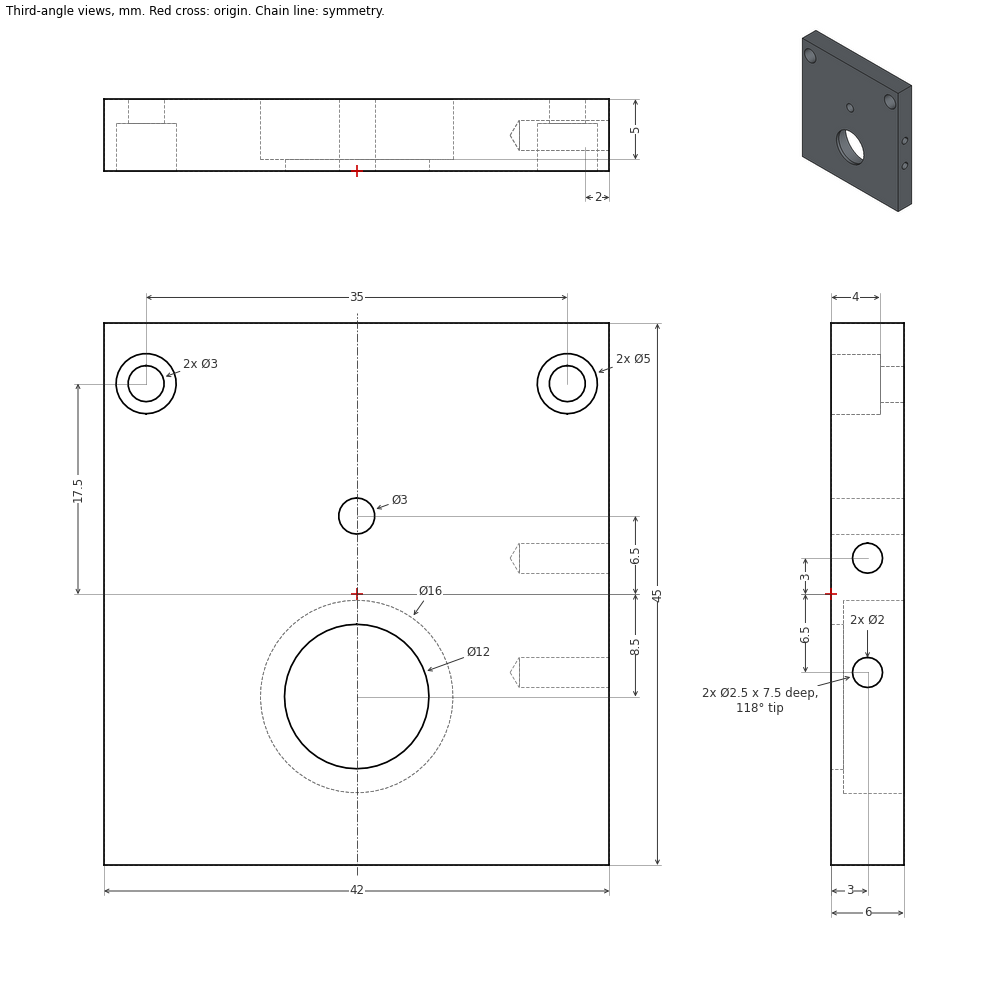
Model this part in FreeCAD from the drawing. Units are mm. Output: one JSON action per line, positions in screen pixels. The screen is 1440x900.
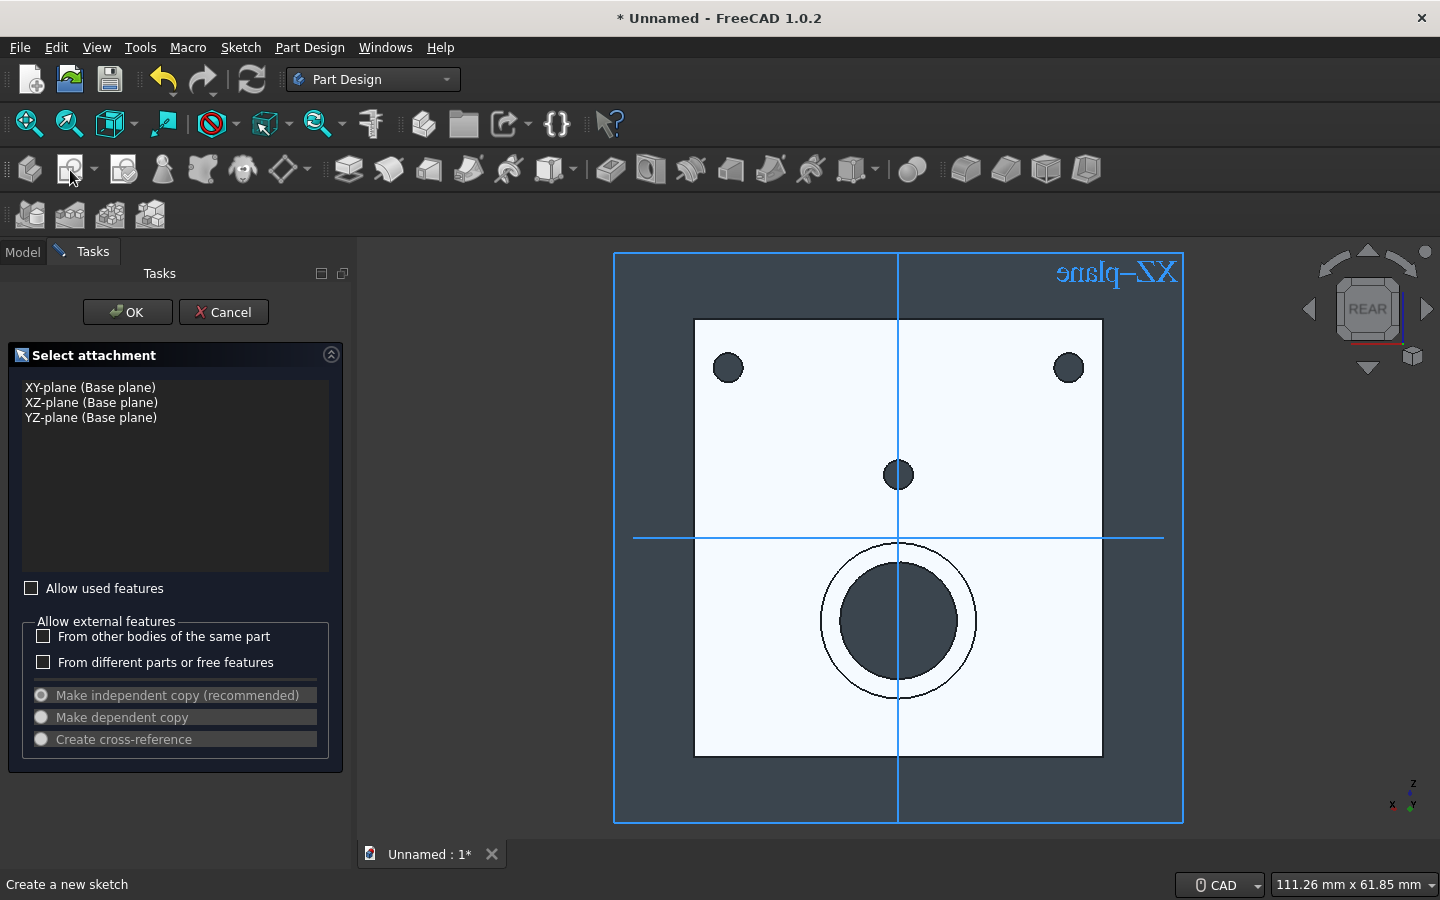
{"action": "left_click", "coordinate": [82, 402]}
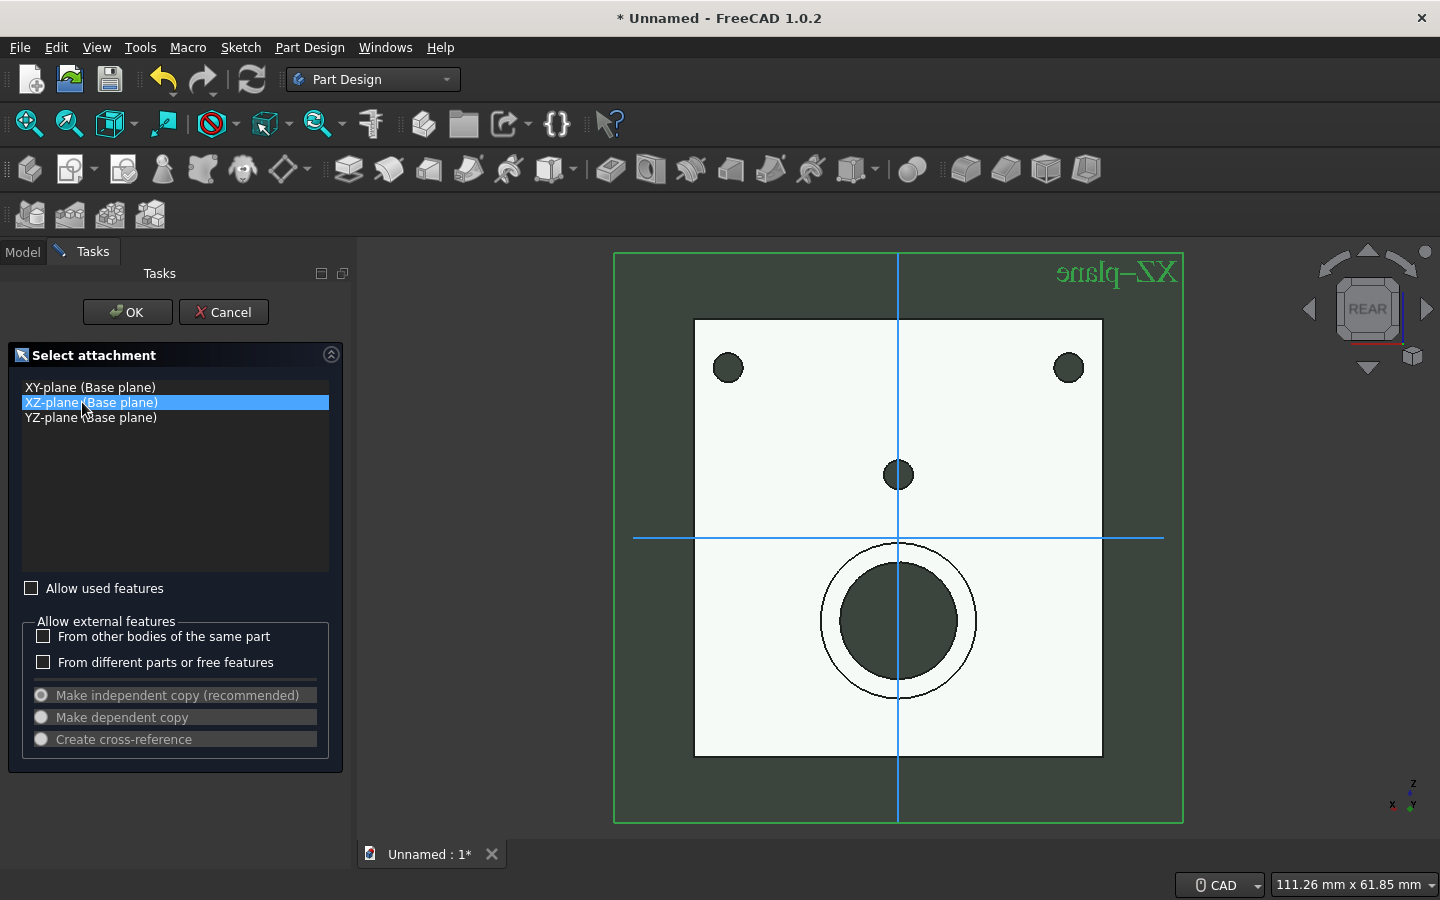
{"action": "left_click", "coordinate": [128, 312]}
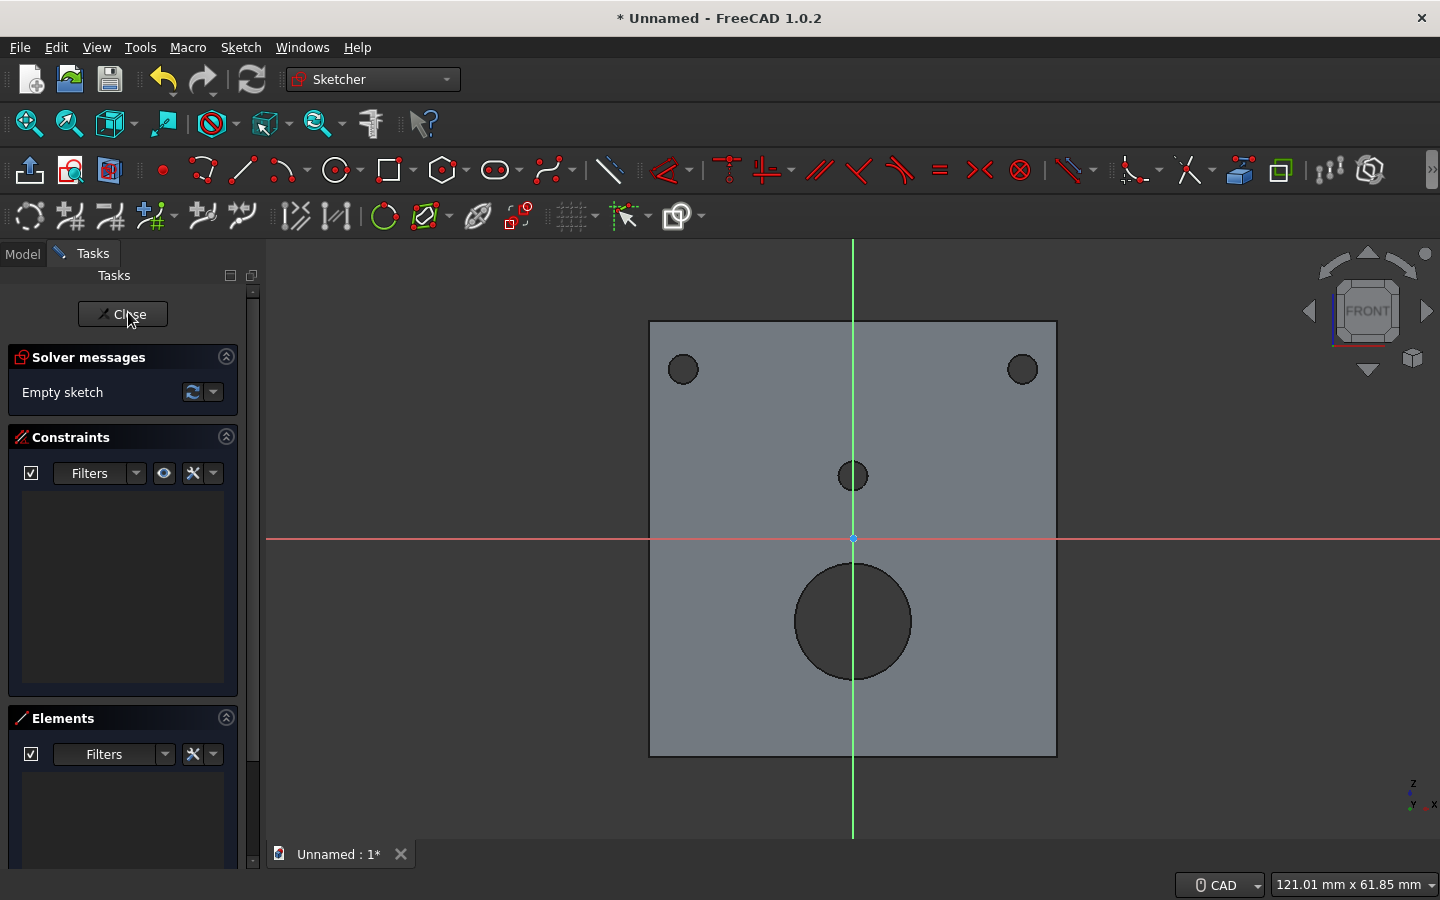
{"action": "scroll", "coordinate": [936, 324], "scroll_direction": "up", "scroll_amount": 3}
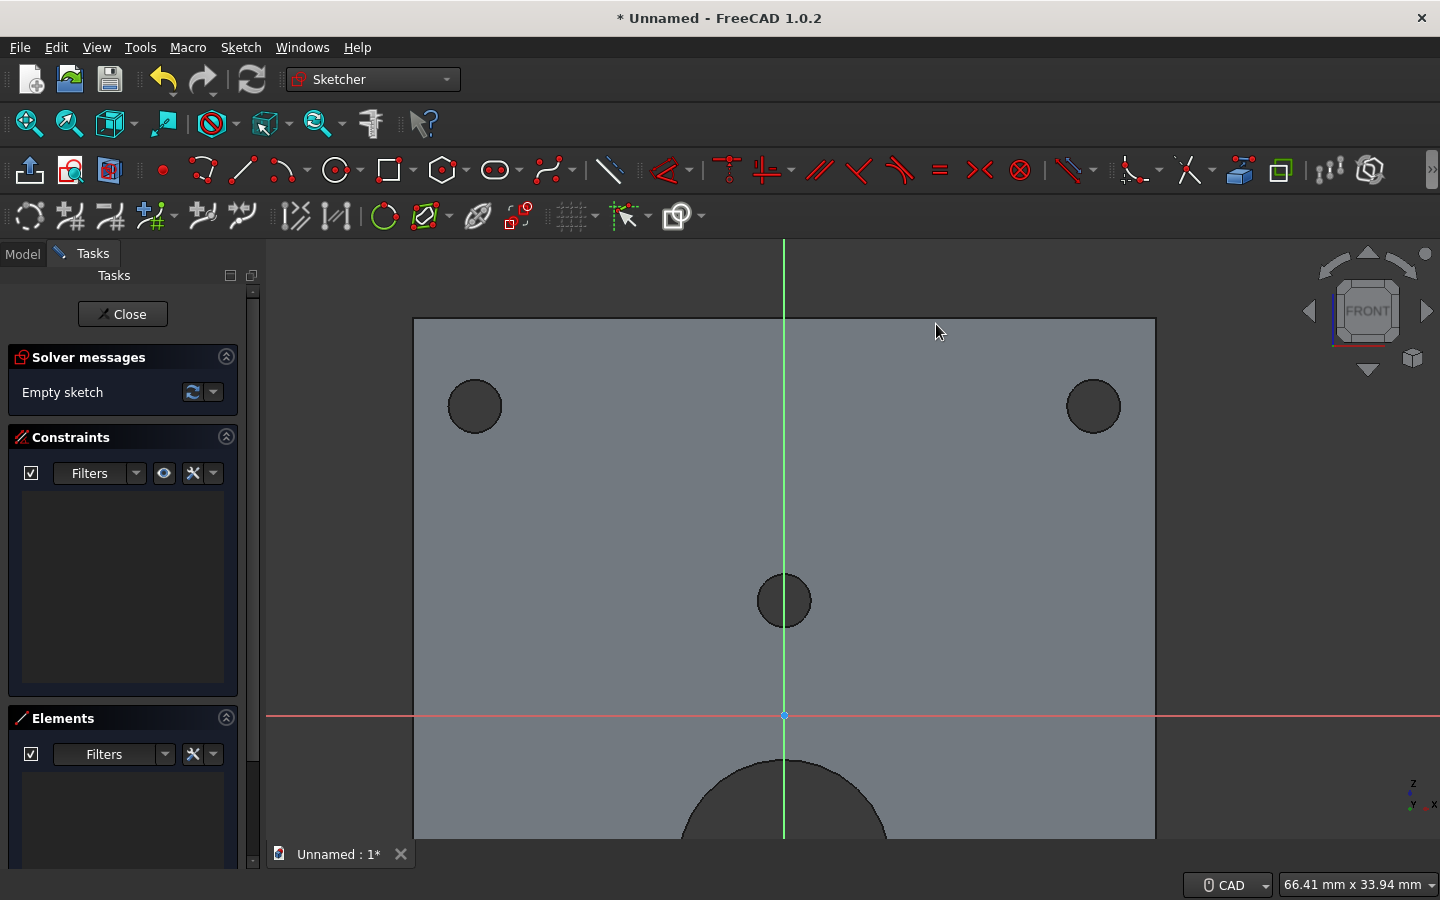
{"action": "key", "text": "g c"}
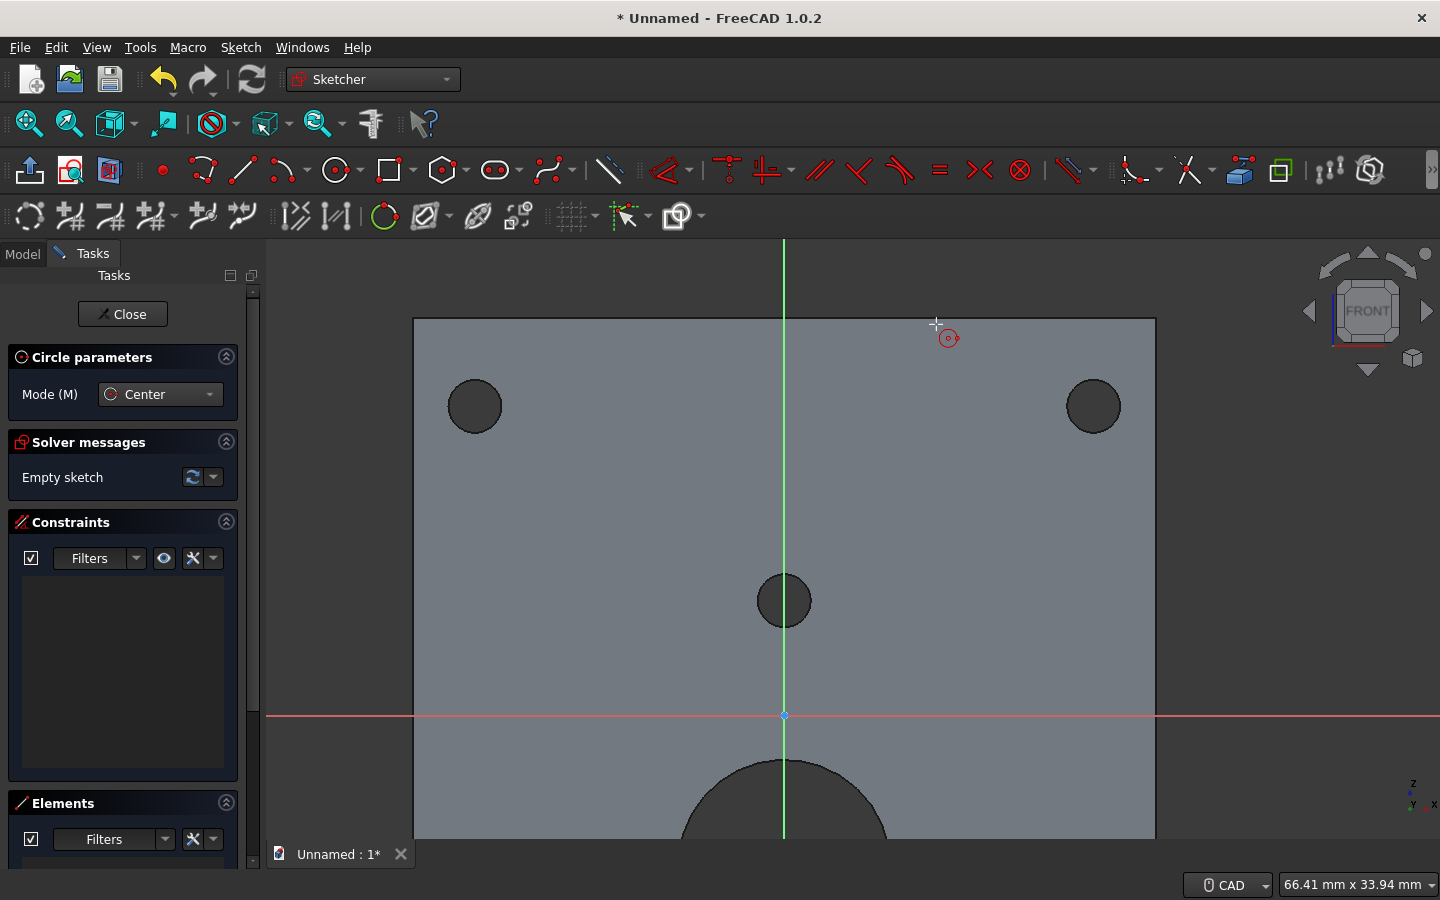
{"action": "left_click", "coordinate": [1094, 406]}
{"action": "mouse_move", "coordinate": [1125, 375]}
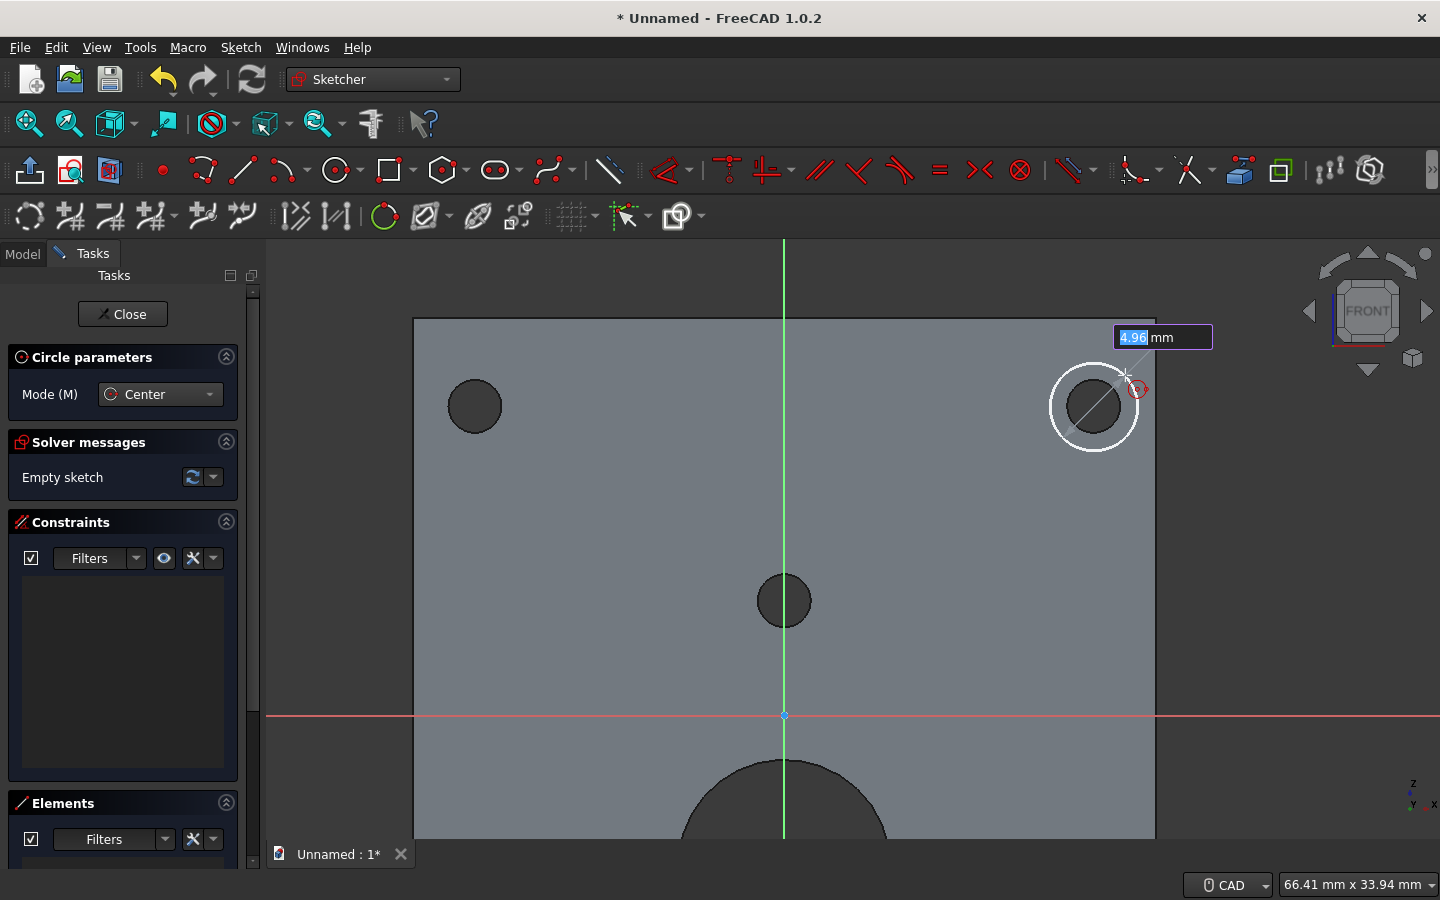
{"action": "type", "text": "5"}
{"action": "key", "text": "Return"}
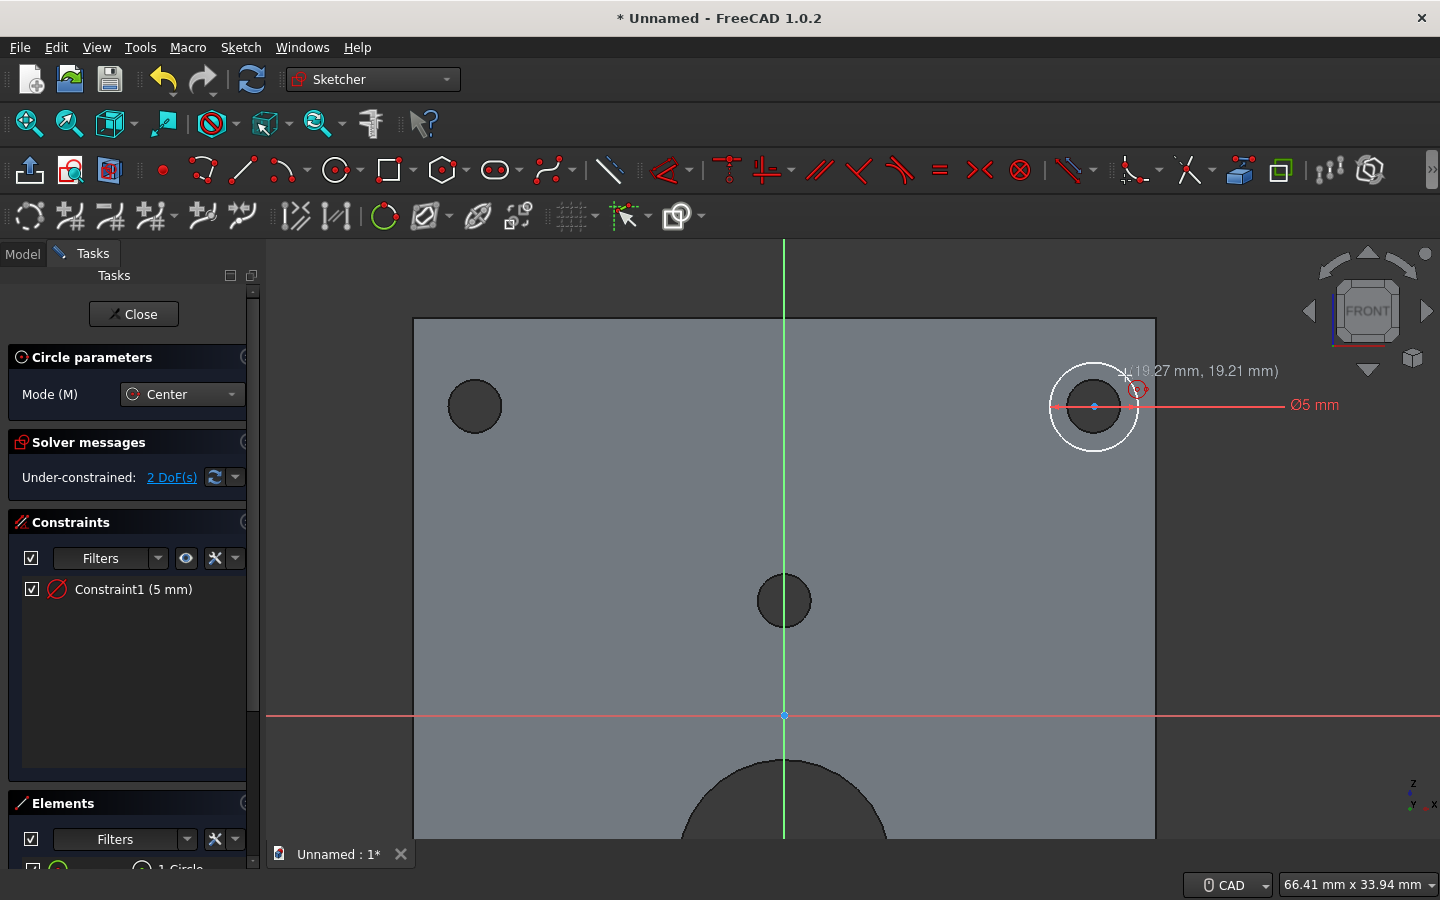
{"action": "left_click", "coordinate": [475, 406]}
{"action": "mouse_move", "coordinate": [506, 375]}